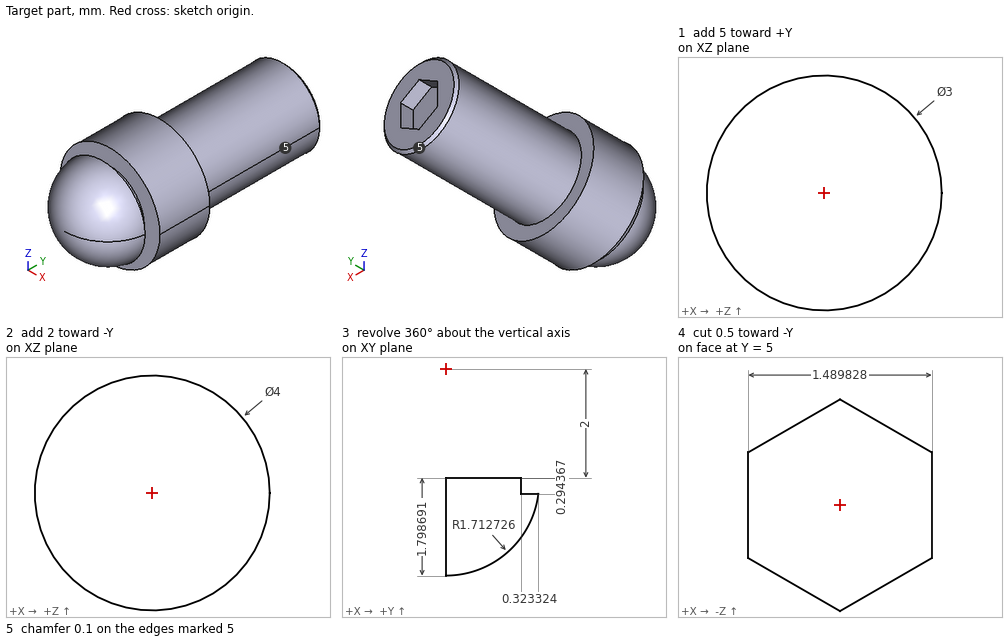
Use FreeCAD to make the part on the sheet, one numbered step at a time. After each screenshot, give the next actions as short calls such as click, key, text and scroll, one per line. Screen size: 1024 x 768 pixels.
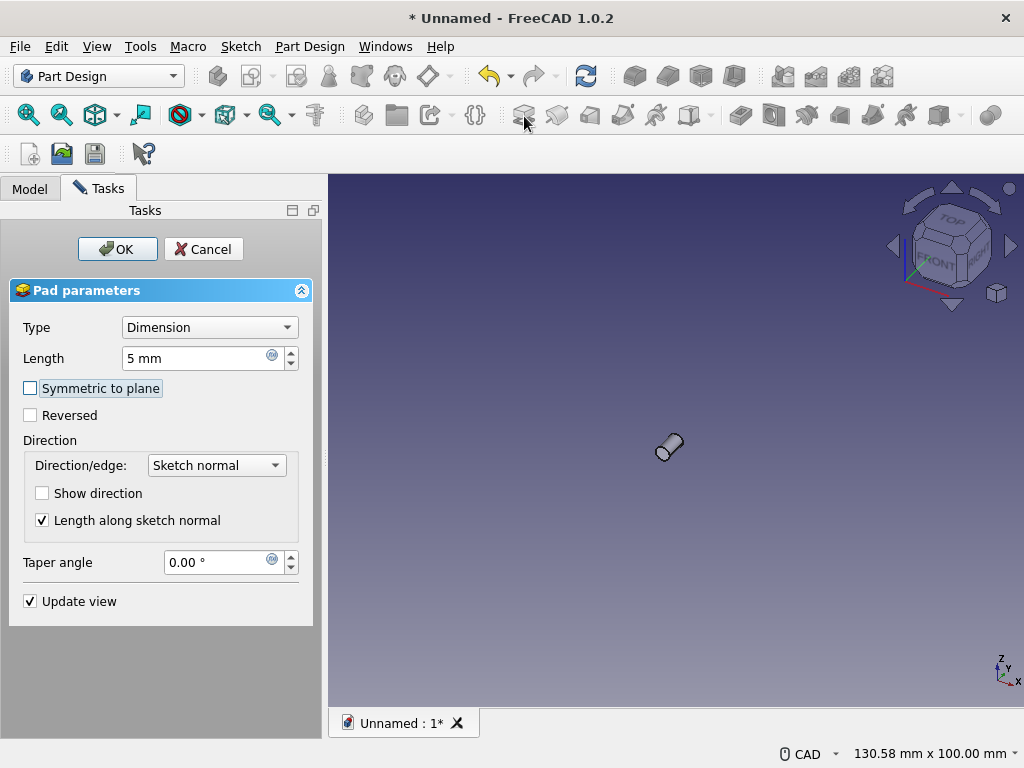
click(31, 415)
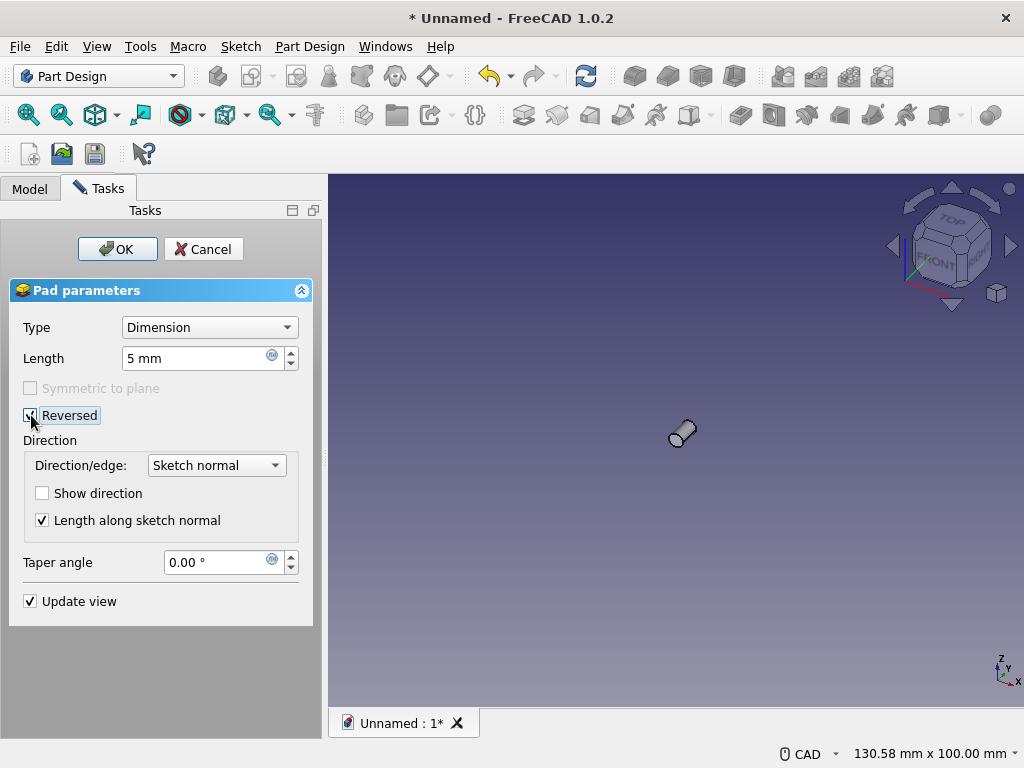
click(118, 249)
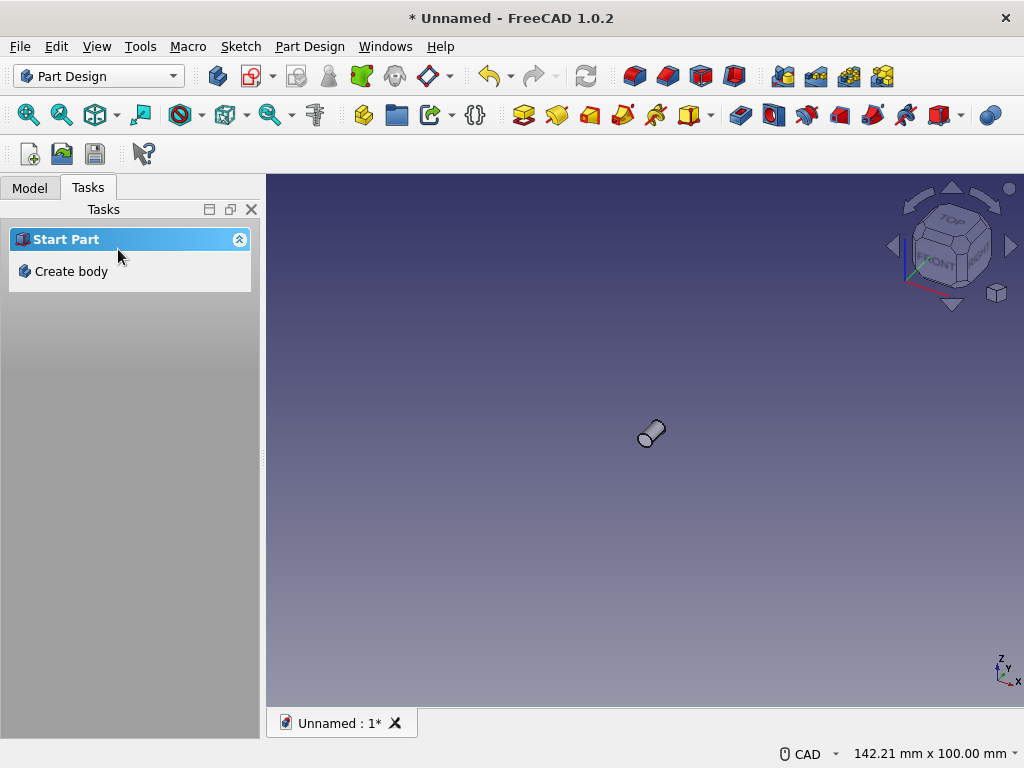
click(29, 116)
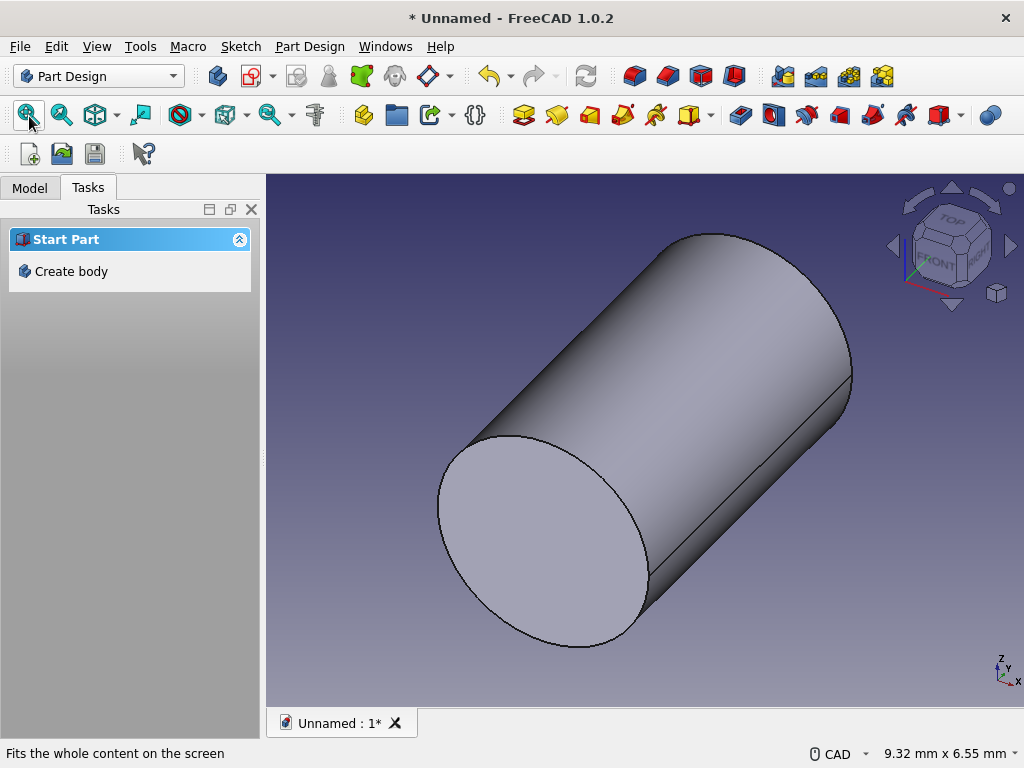
click(250, 76)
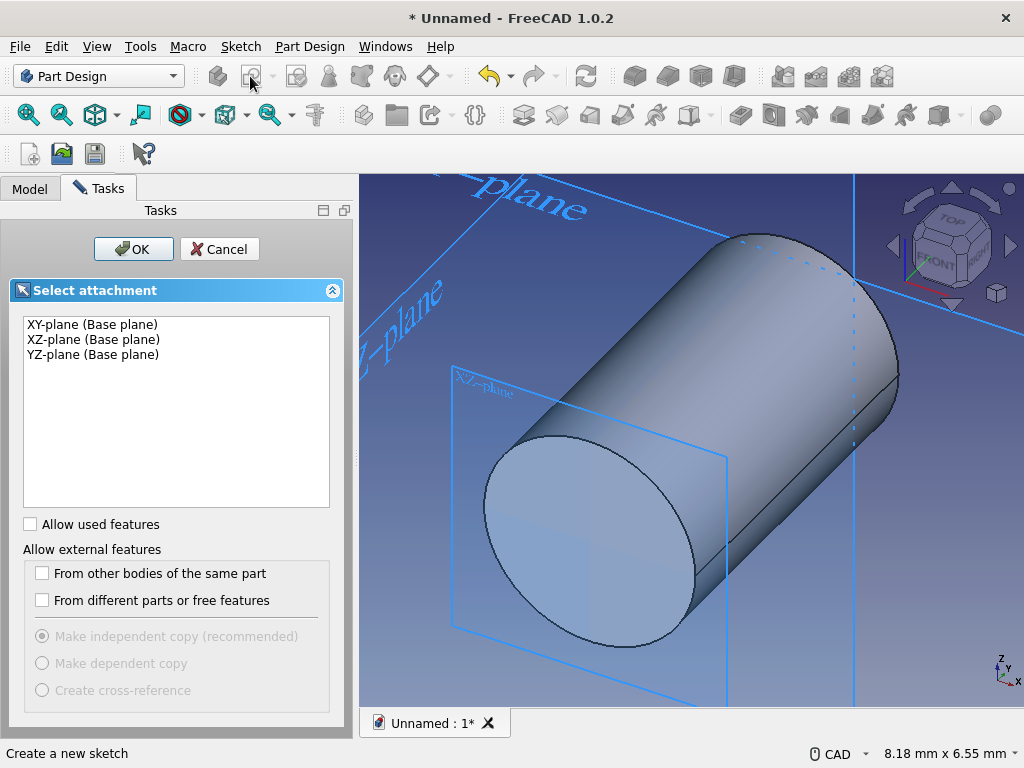
click(84, 340)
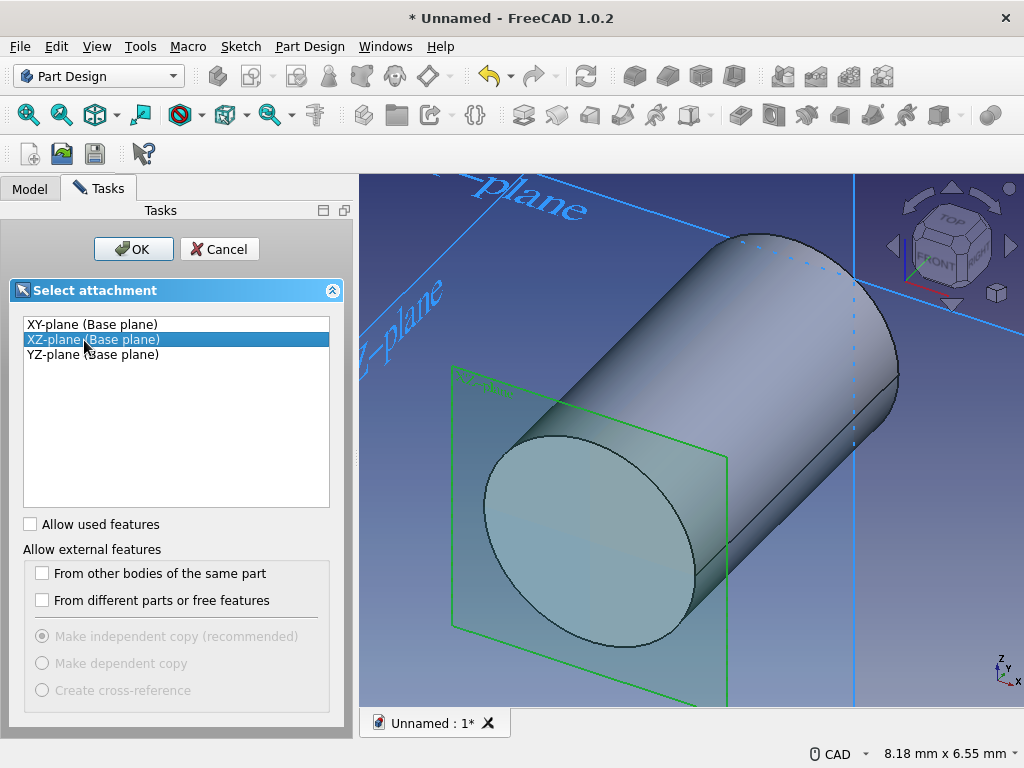
click(134, 249)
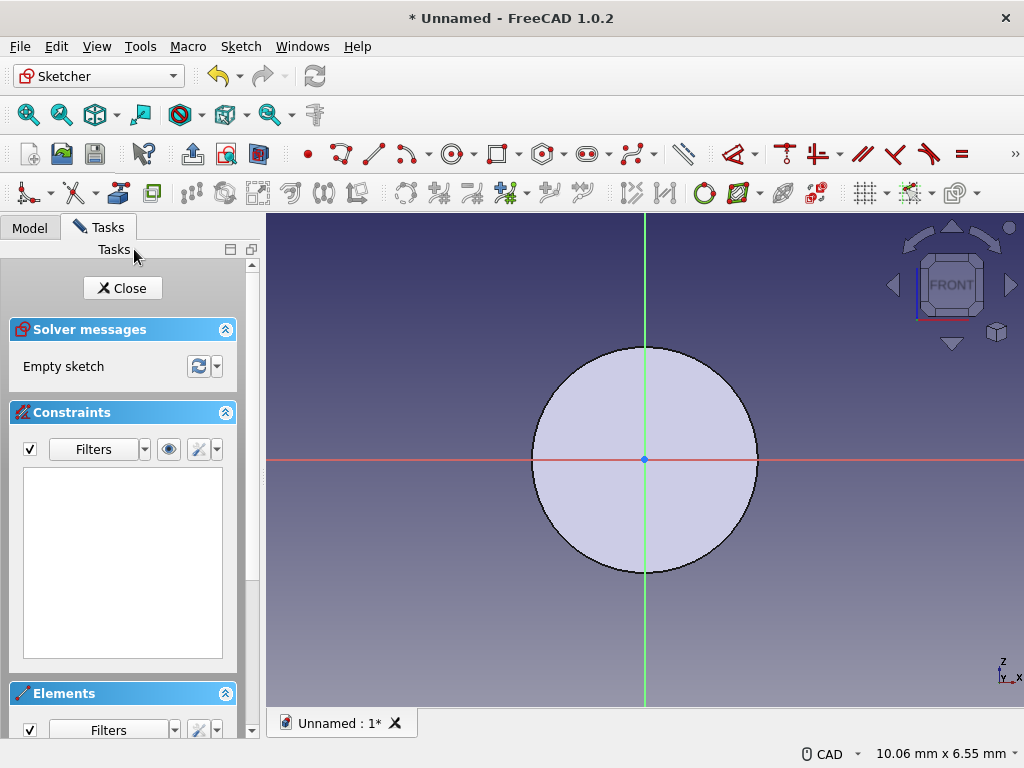
click(452, 154)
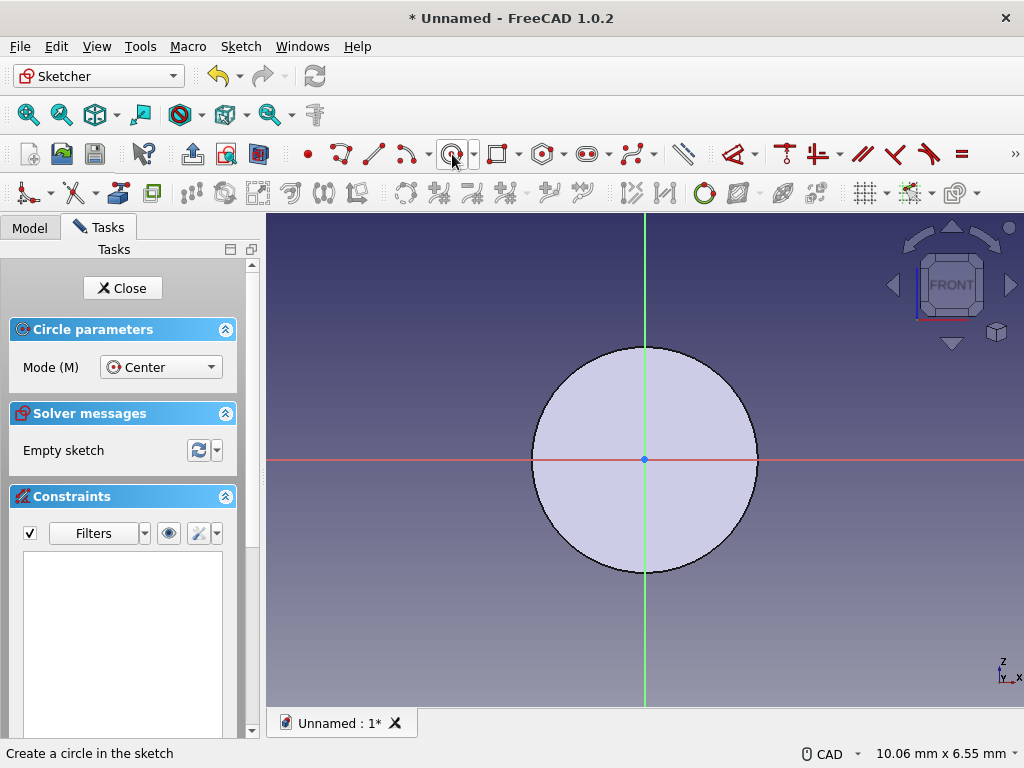
click(645, 460)
click(751, 353)
key(Escape)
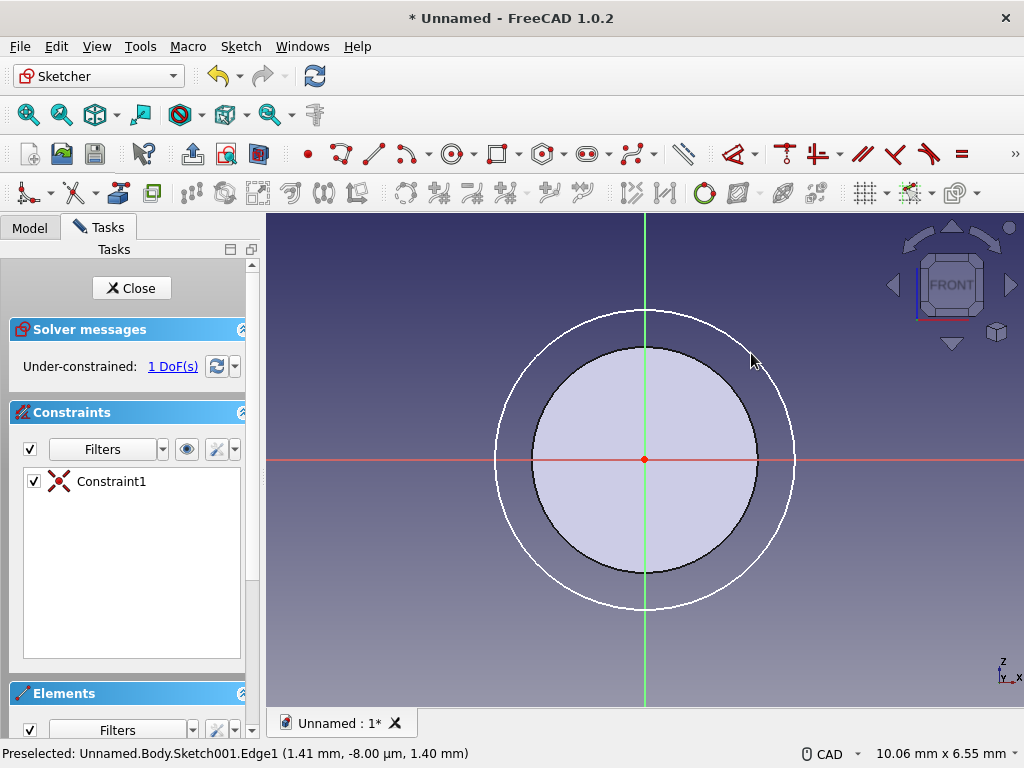
click(751, 354)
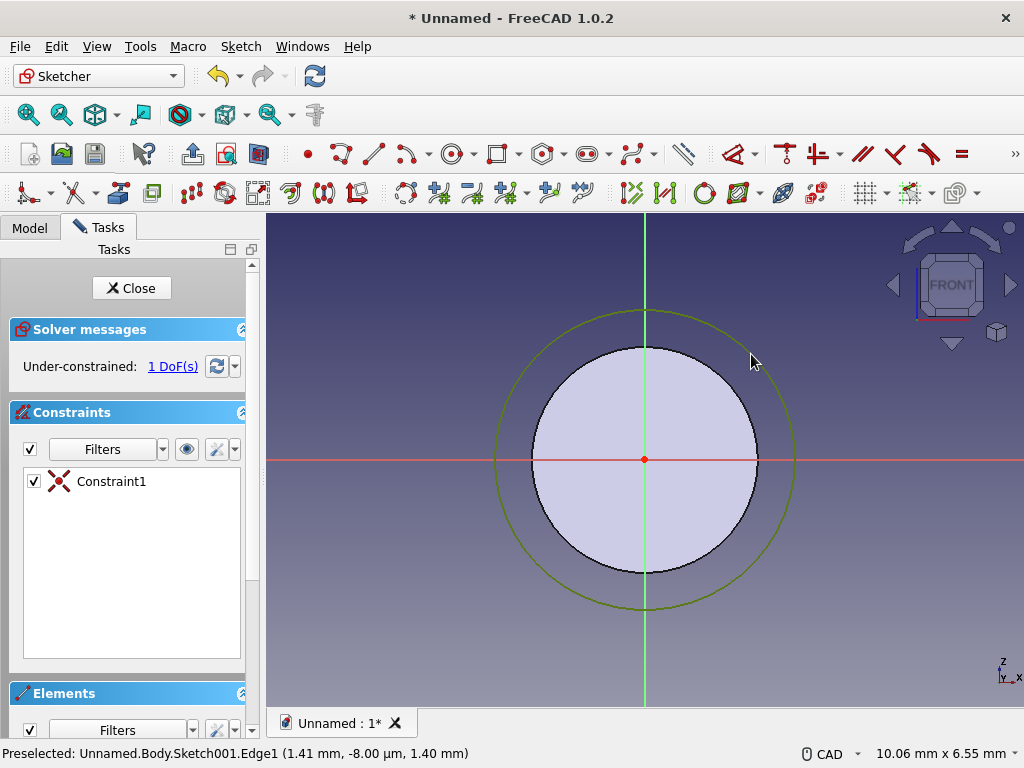
click(754, 154)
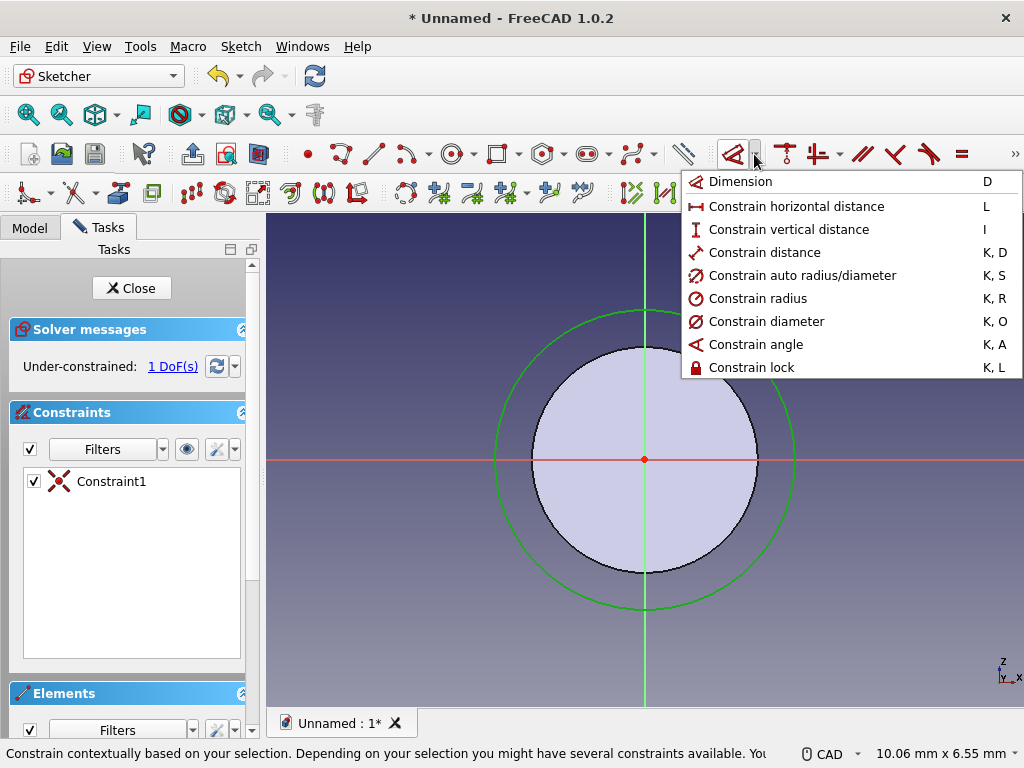
click(852, 322)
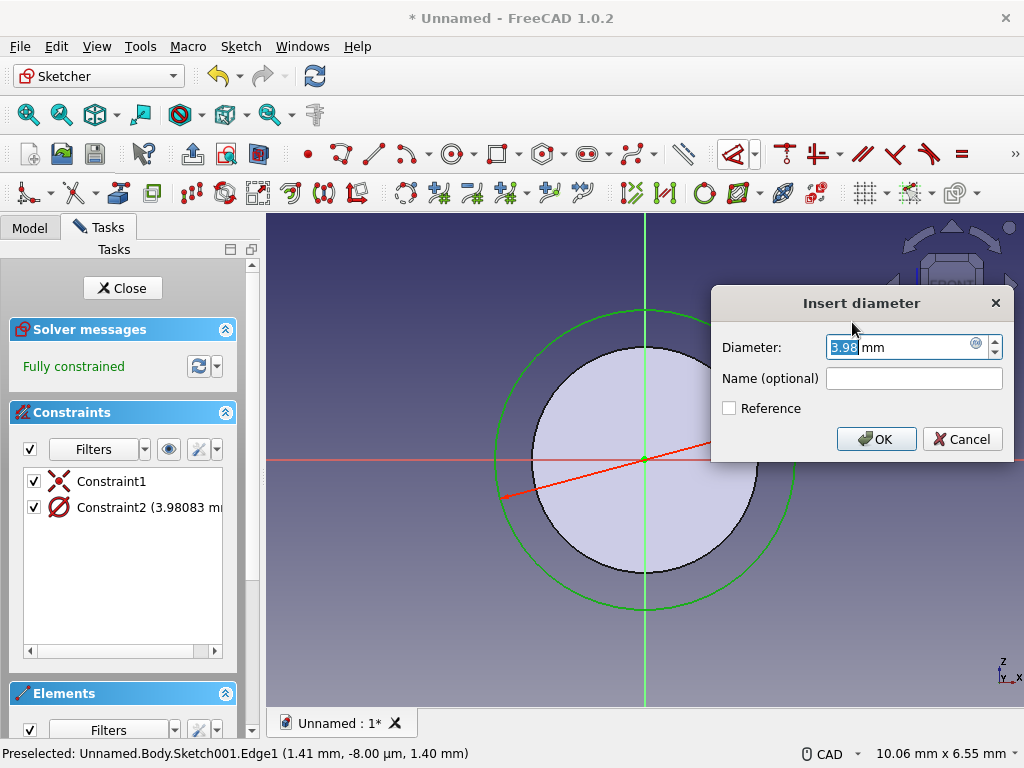
text(4)
key(Return)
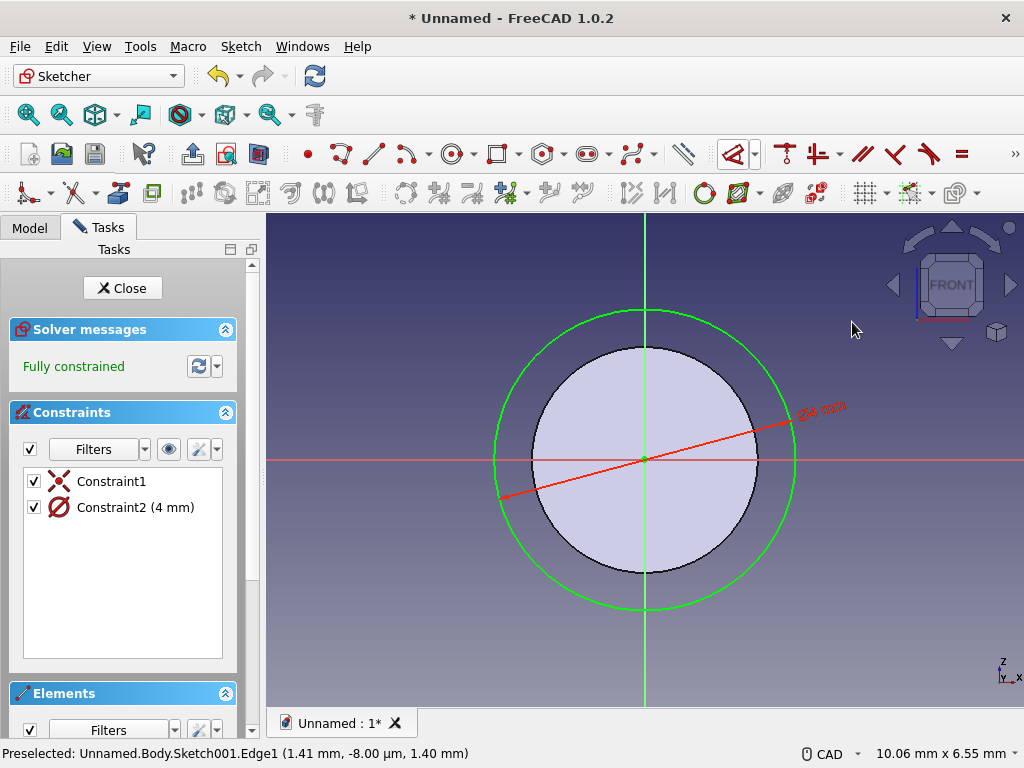
click(123, 288)